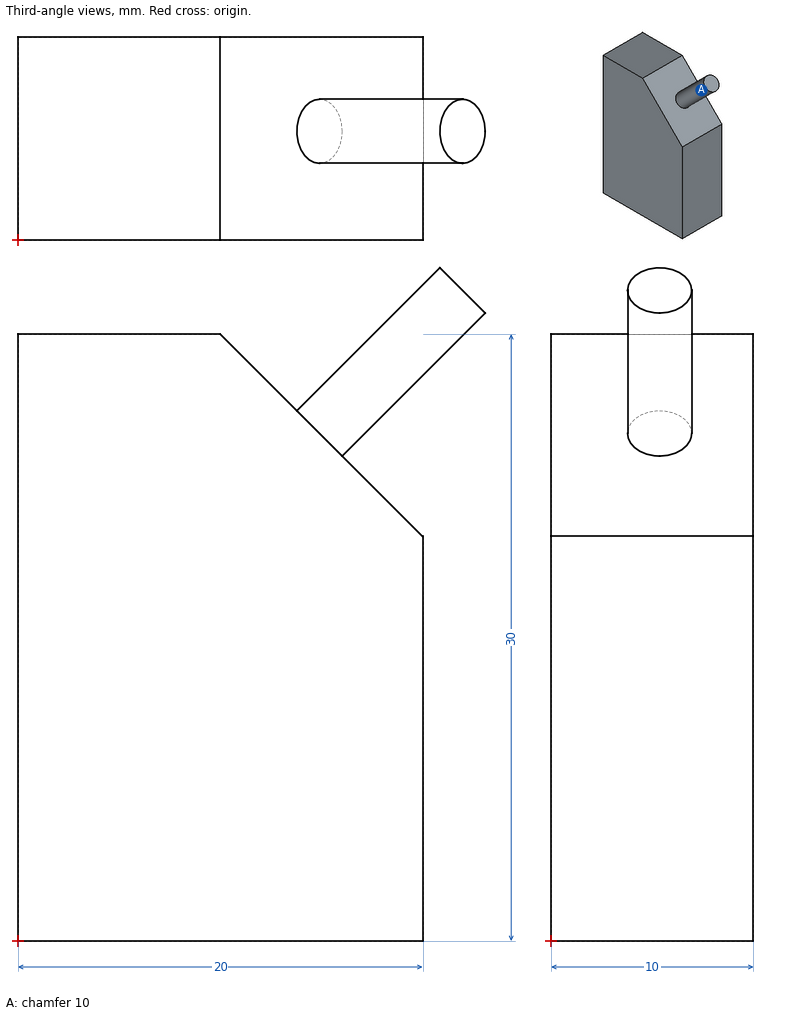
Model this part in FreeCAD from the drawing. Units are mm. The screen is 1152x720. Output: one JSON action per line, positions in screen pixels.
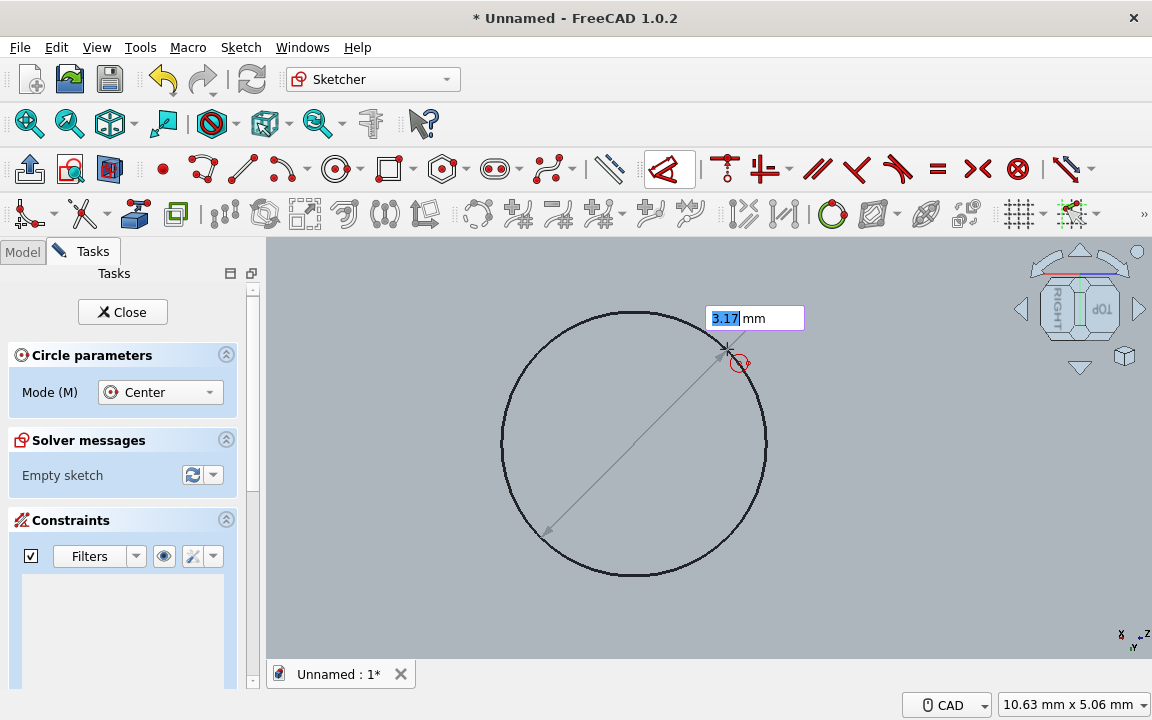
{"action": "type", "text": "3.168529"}
{"action": "key", "text": "Return"}
{"action": "key", "text": "Escape"}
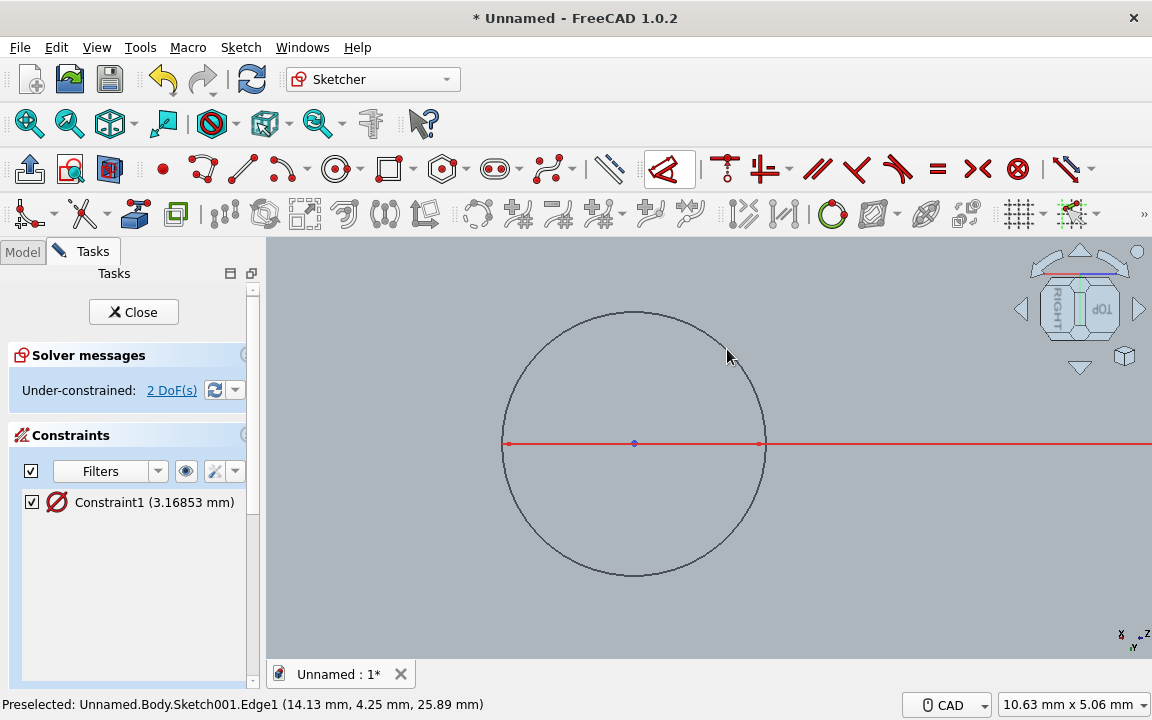
{"action": "key", "text": "d"}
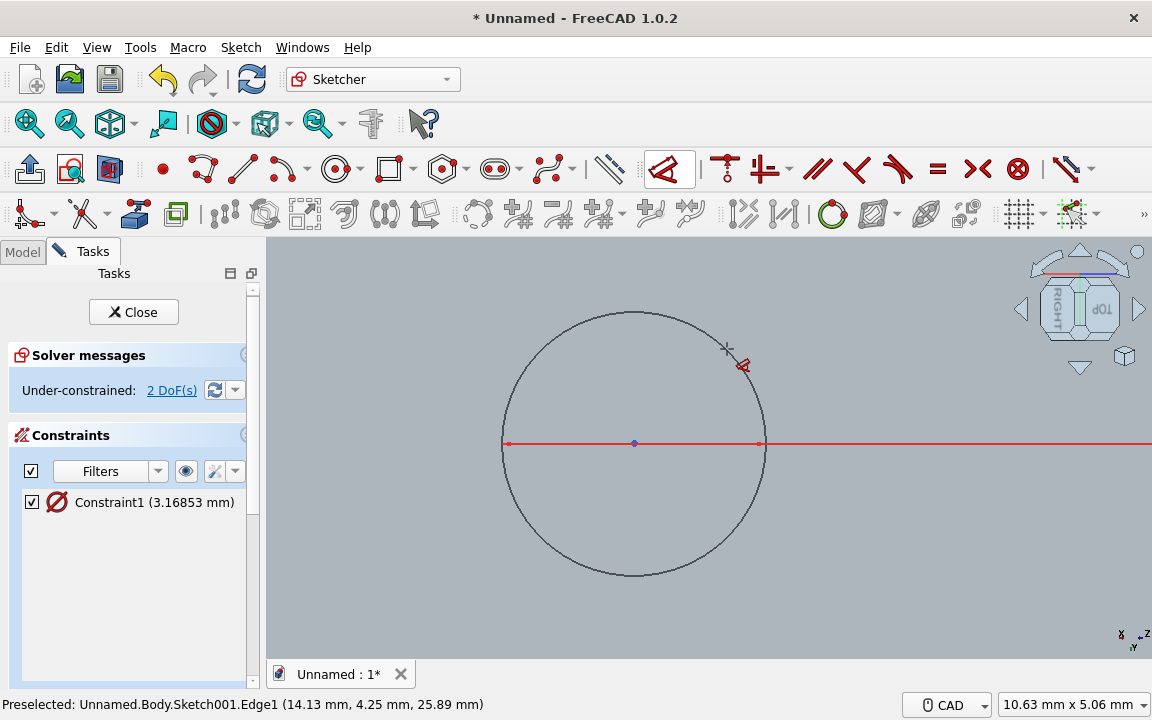
{"action": "left_click", "coordinate": [634, 444]}
{"action": "left_click", "coordinate": [464, 478]}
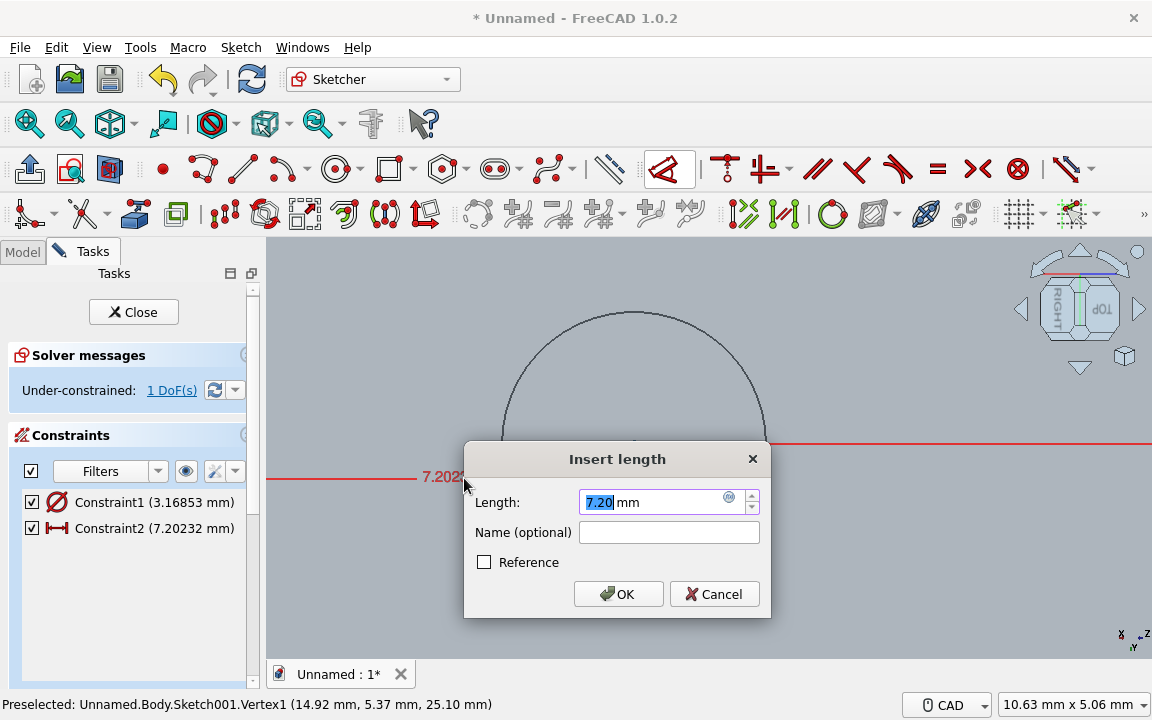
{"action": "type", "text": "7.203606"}
{"action": "key", "text": "Return"}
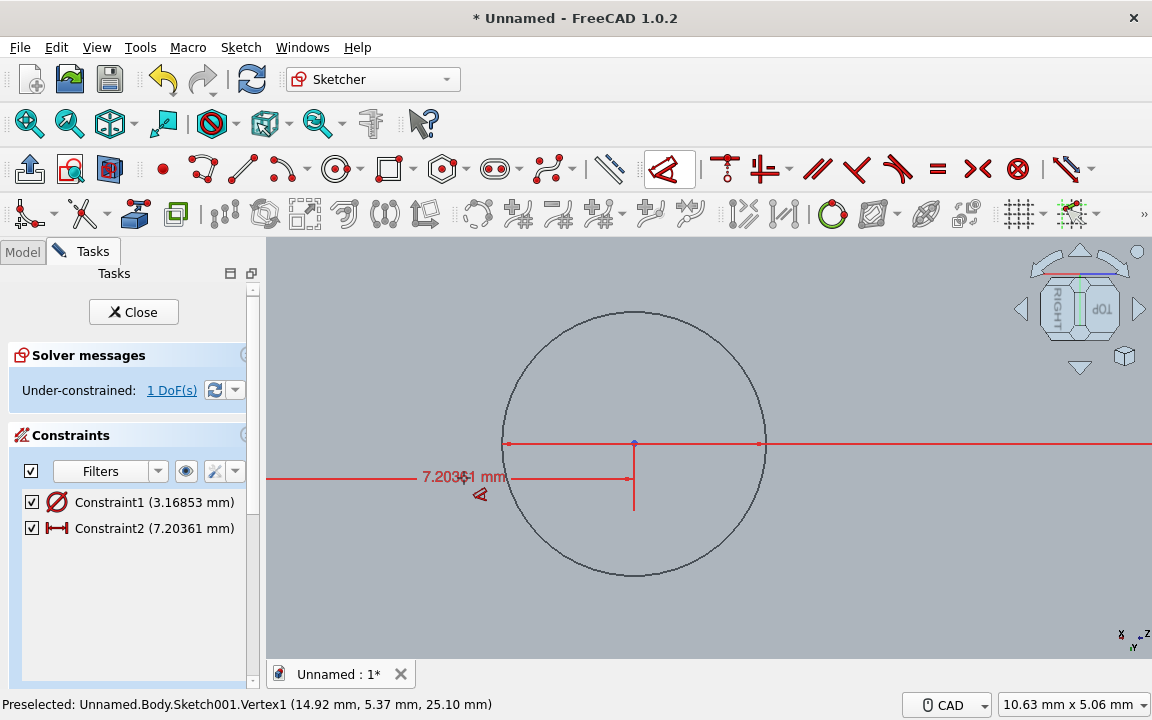
{"action": "left_click", "coordinate": [634, 444]}
{"action": "left_click", "coordinate": [668, 355]}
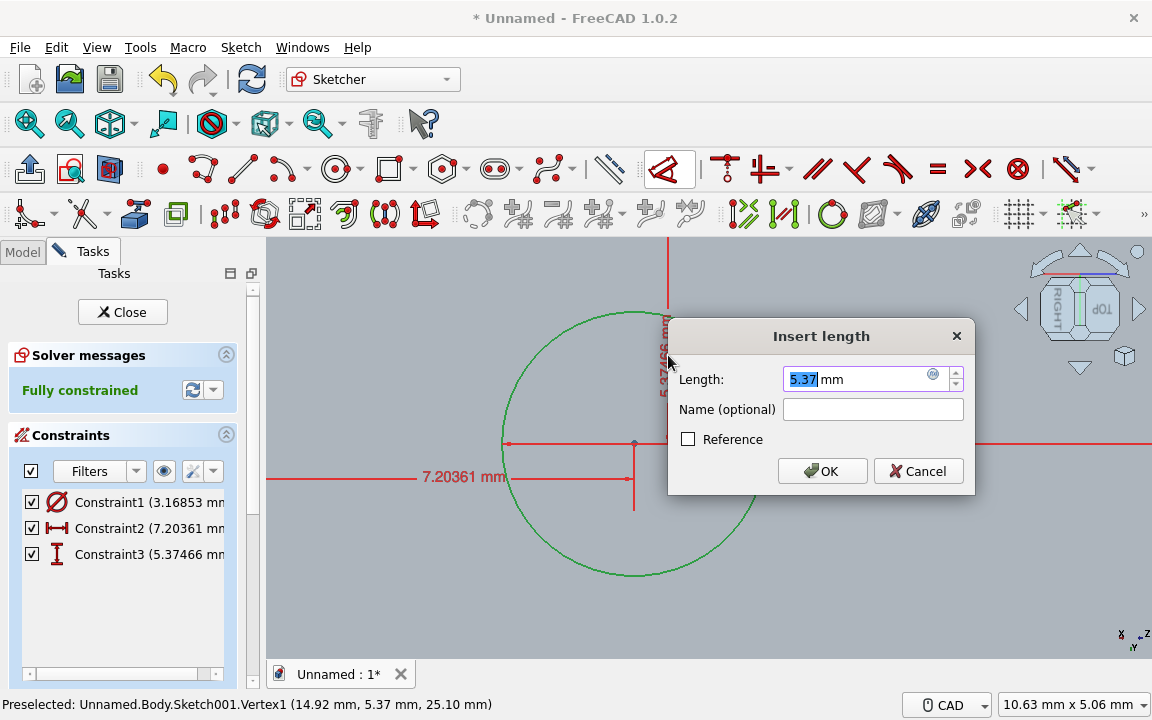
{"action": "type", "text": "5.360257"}
{"action": "key", "text": "Return"}
{"action": "key", "text": "Escape"}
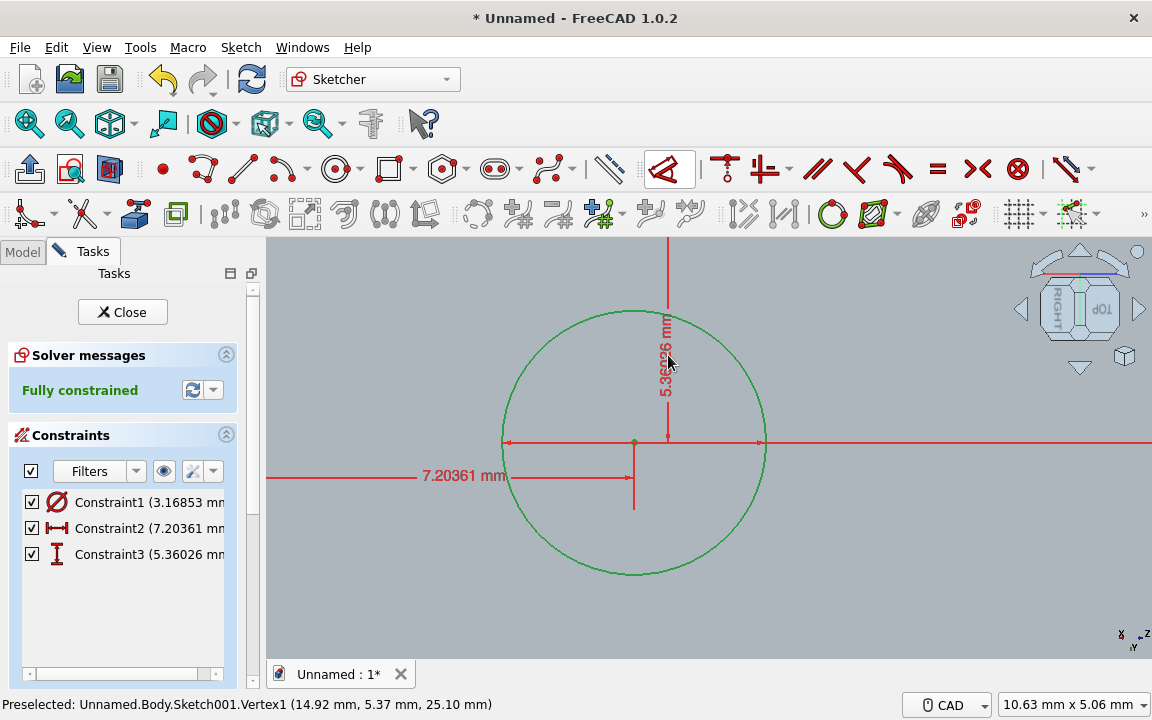
{"action": "left_click", "coordinate": [123, 312]}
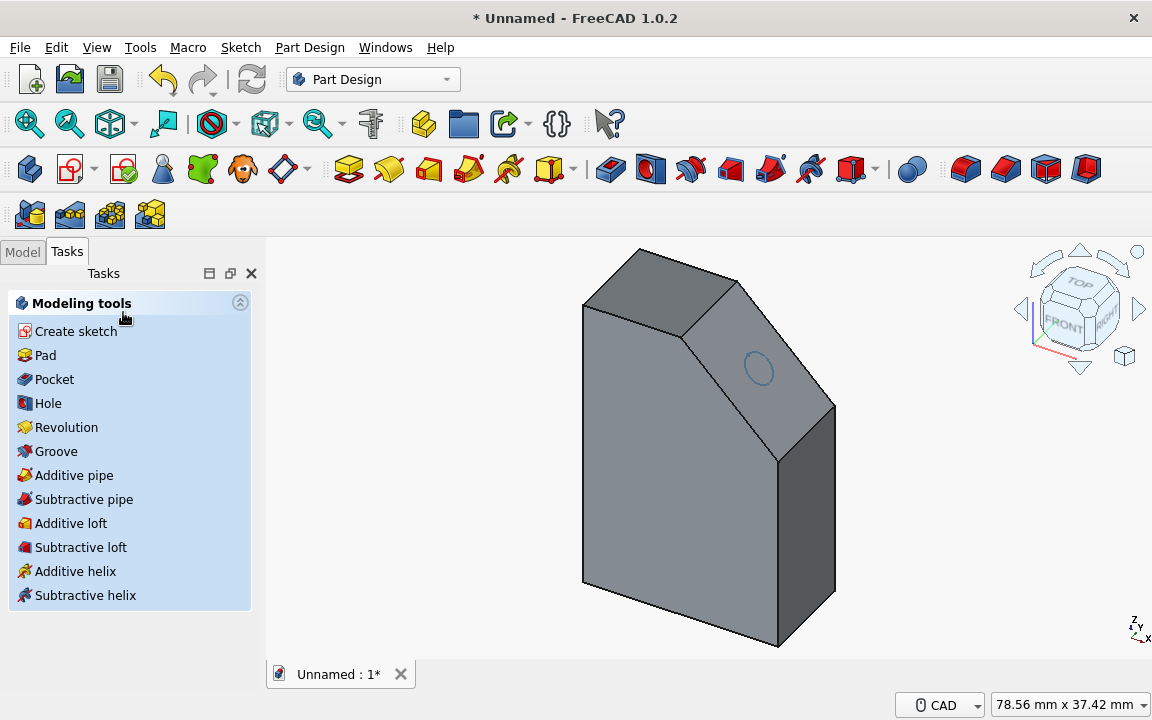
{"action": "left_click", "coordinate": [350, 170]}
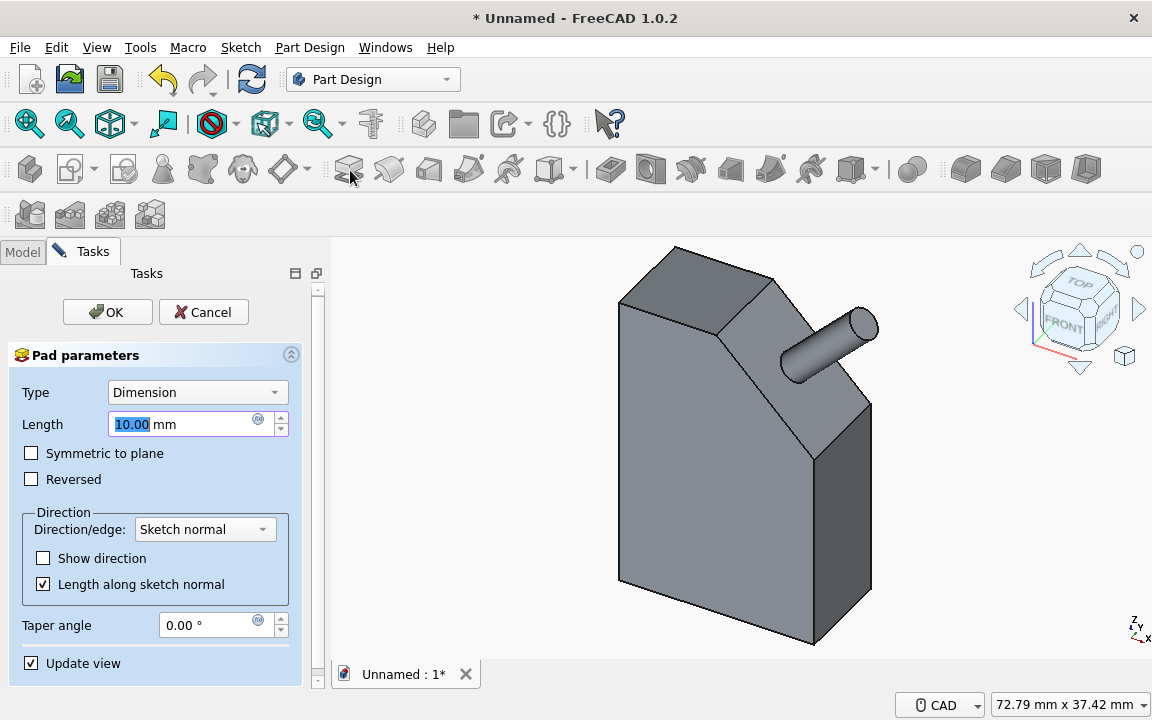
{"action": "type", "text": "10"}
{"action": "key", "text": "Tab"}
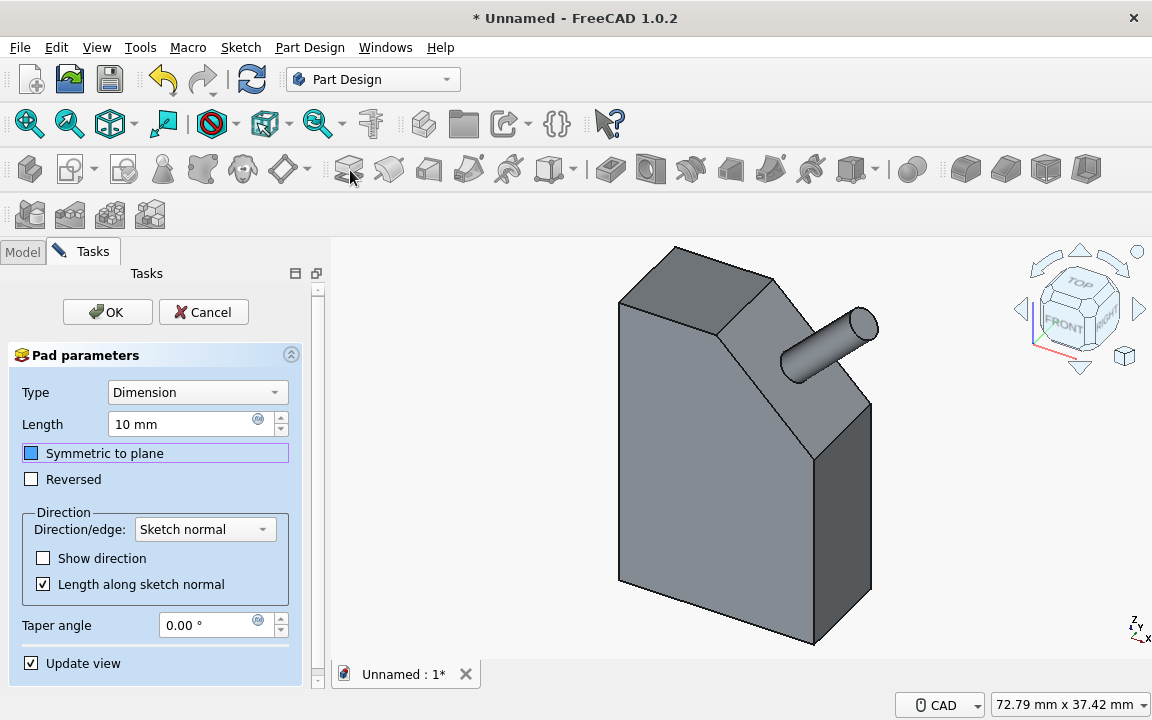
{"action": "left_click", "coordinate": [108, 312]}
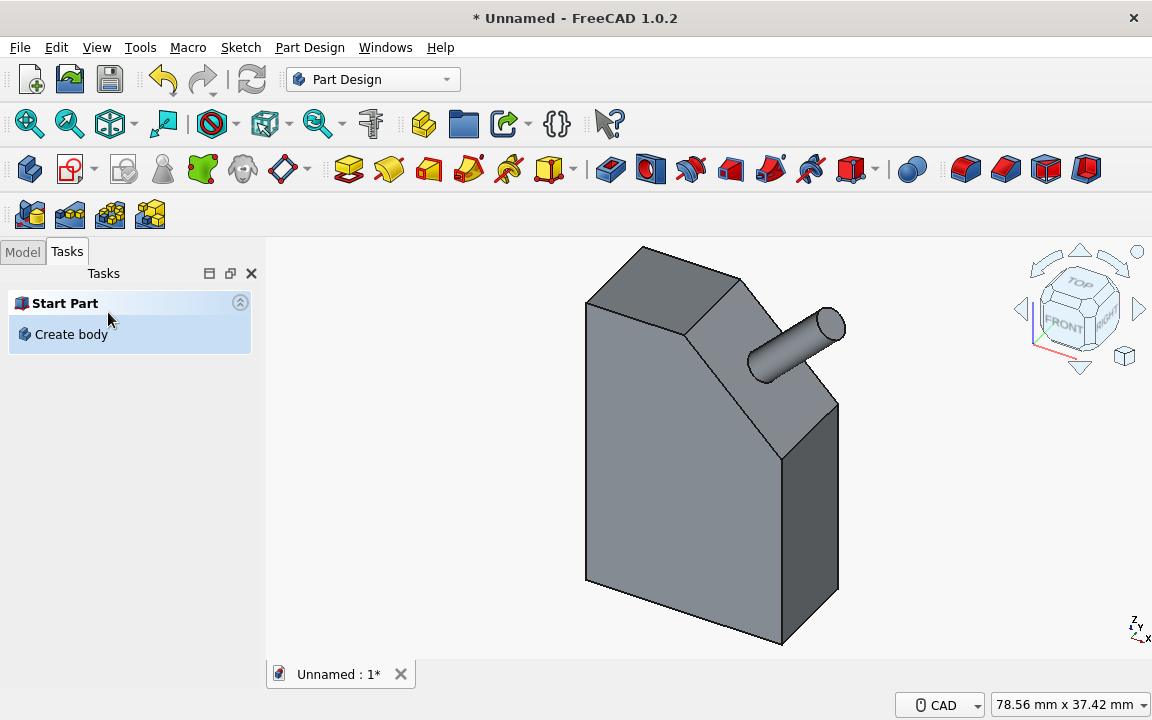
{"action": "key", "text": "0"}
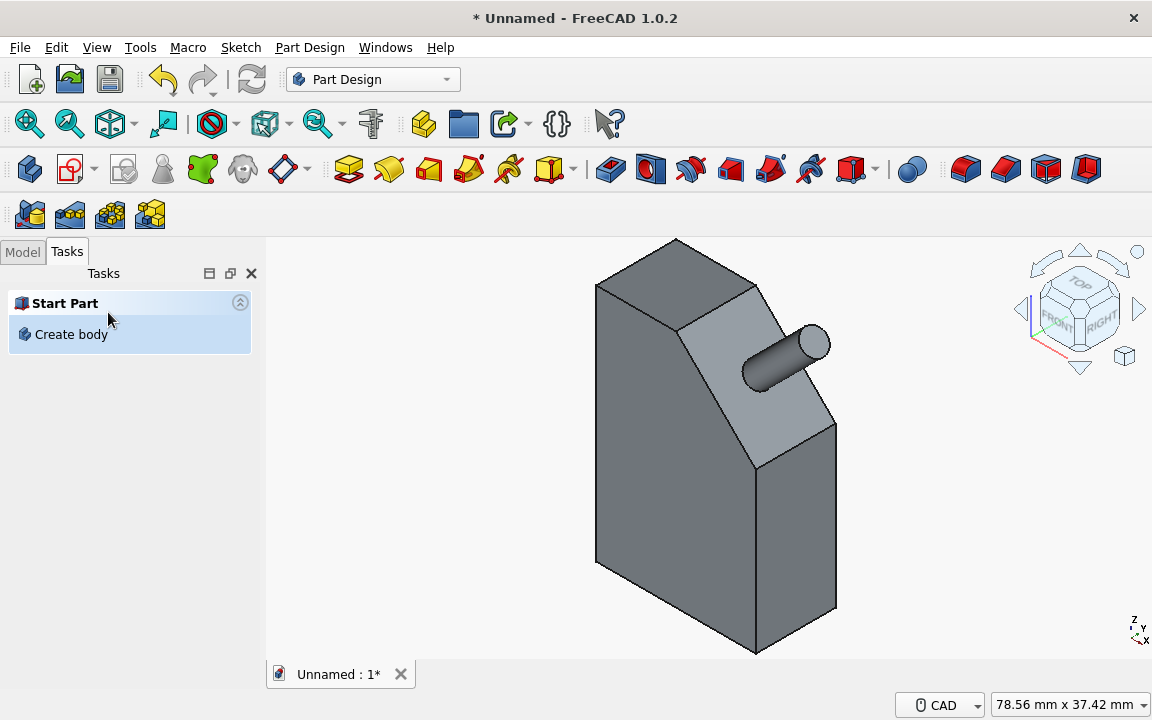
{"action": "key", "text": "v f"}